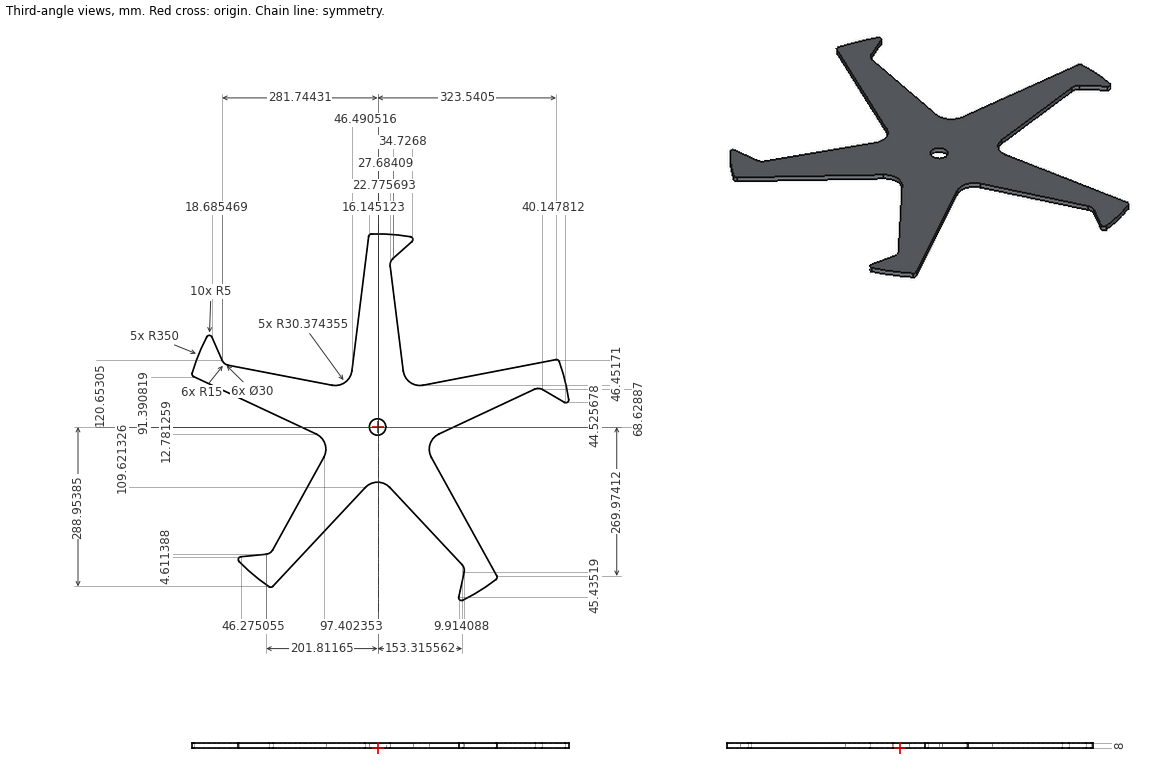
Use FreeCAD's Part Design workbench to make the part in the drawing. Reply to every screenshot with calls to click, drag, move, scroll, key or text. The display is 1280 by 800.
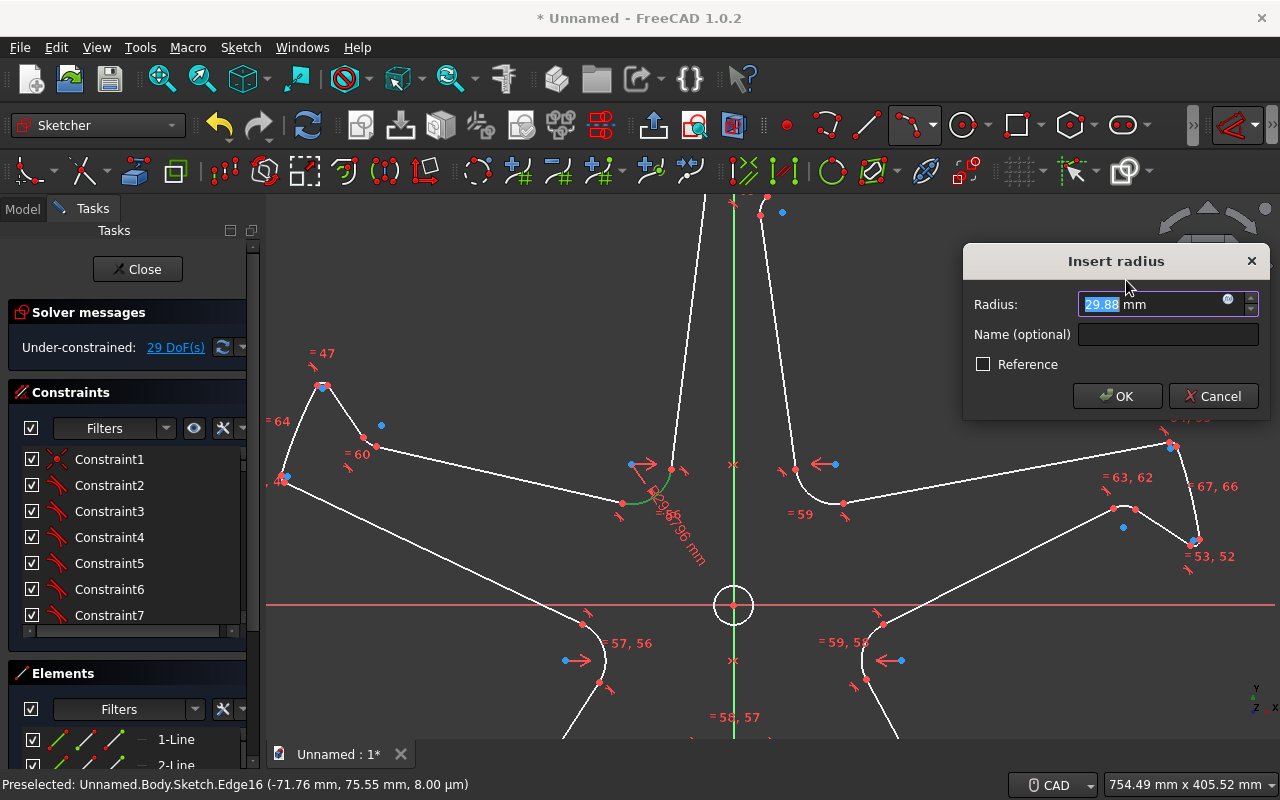
text(30.374355)
key(Return)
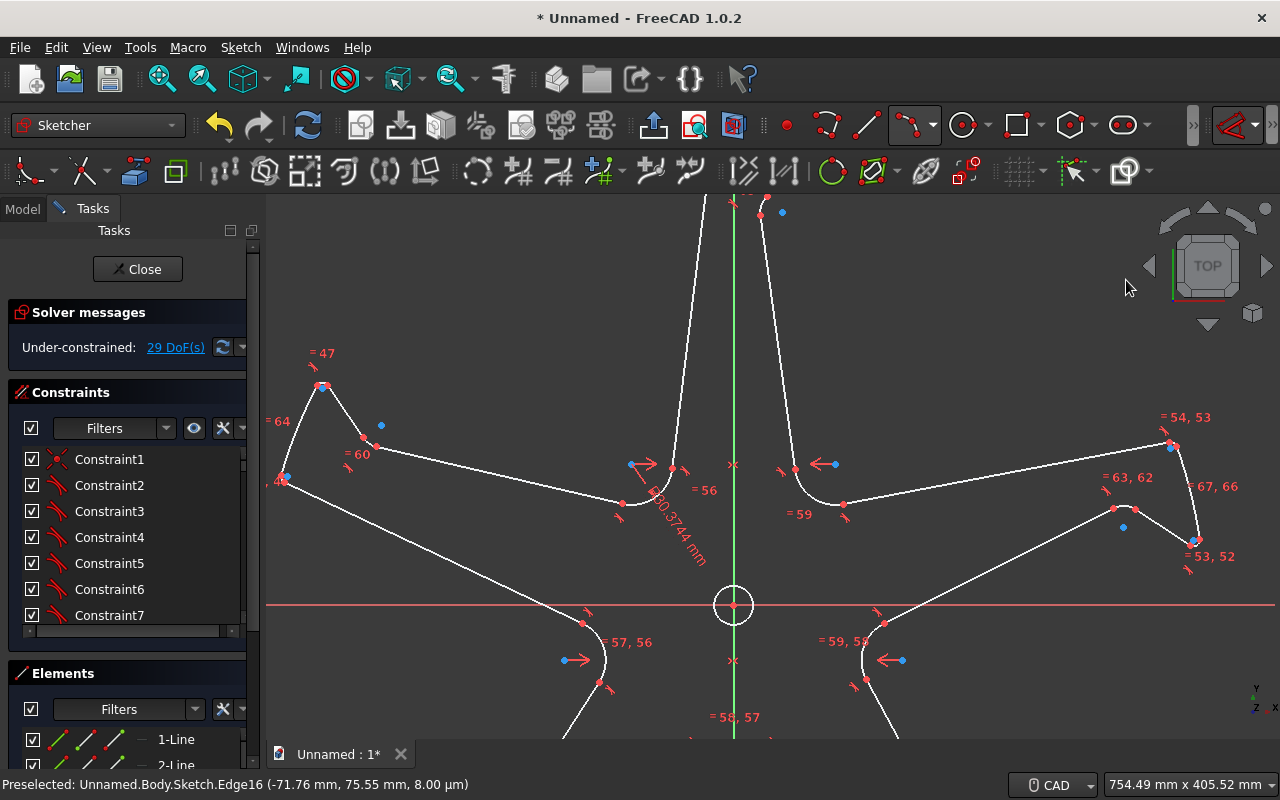
scroll(369, 444, up, 4)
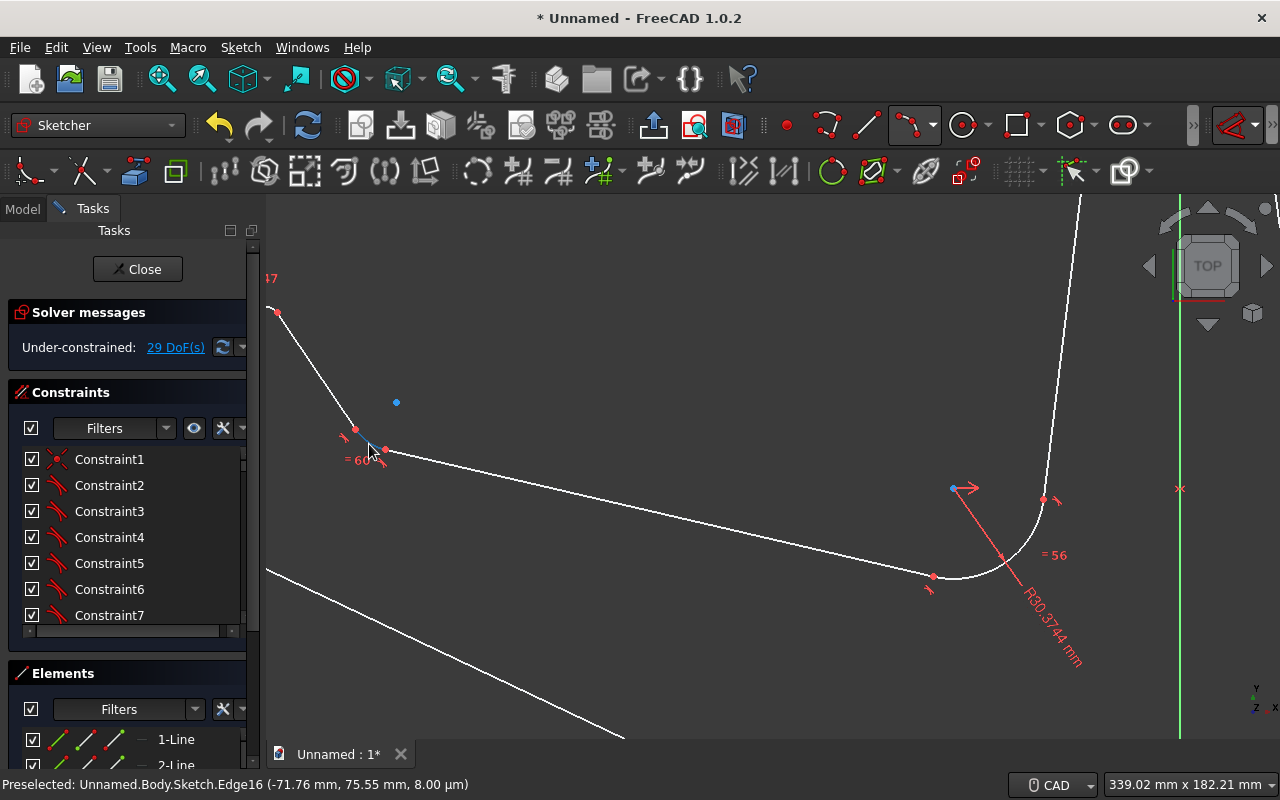
click(369, 442)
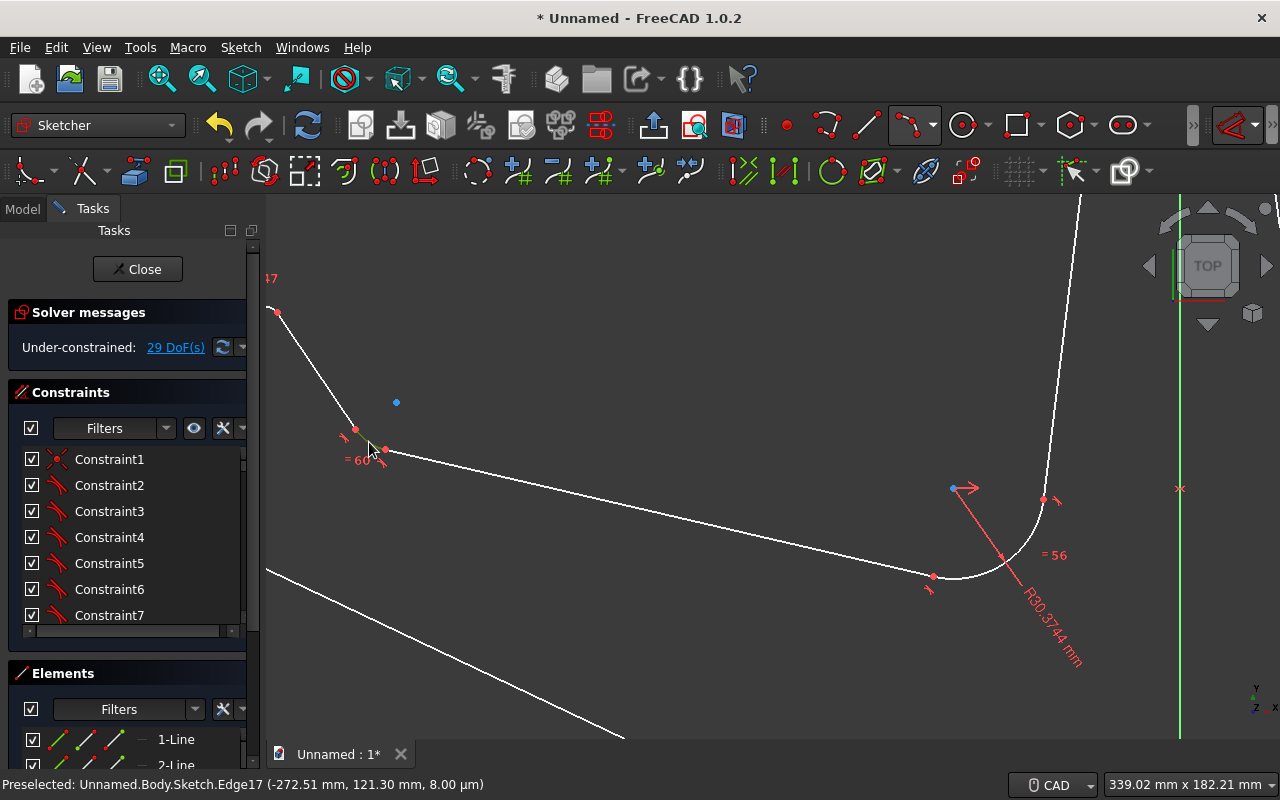
key(k)
key(r)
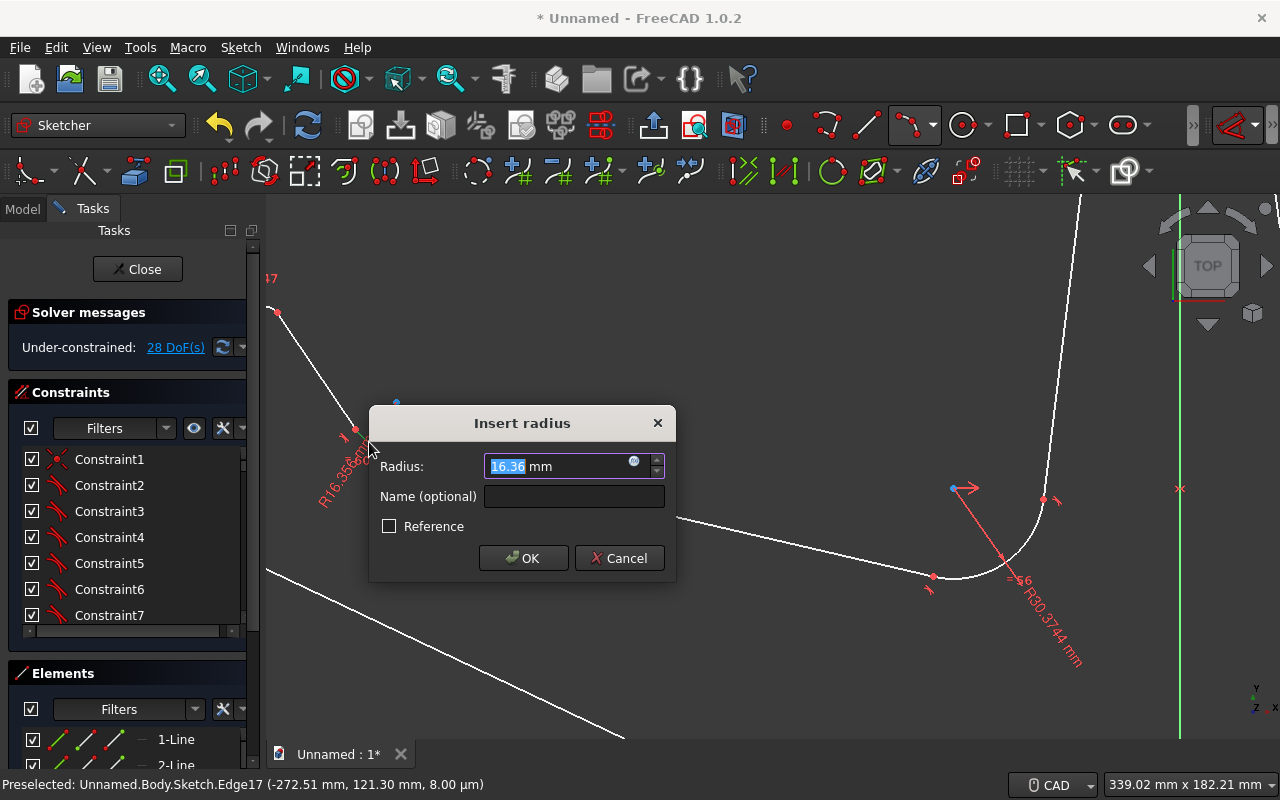
text(15)
key(Return)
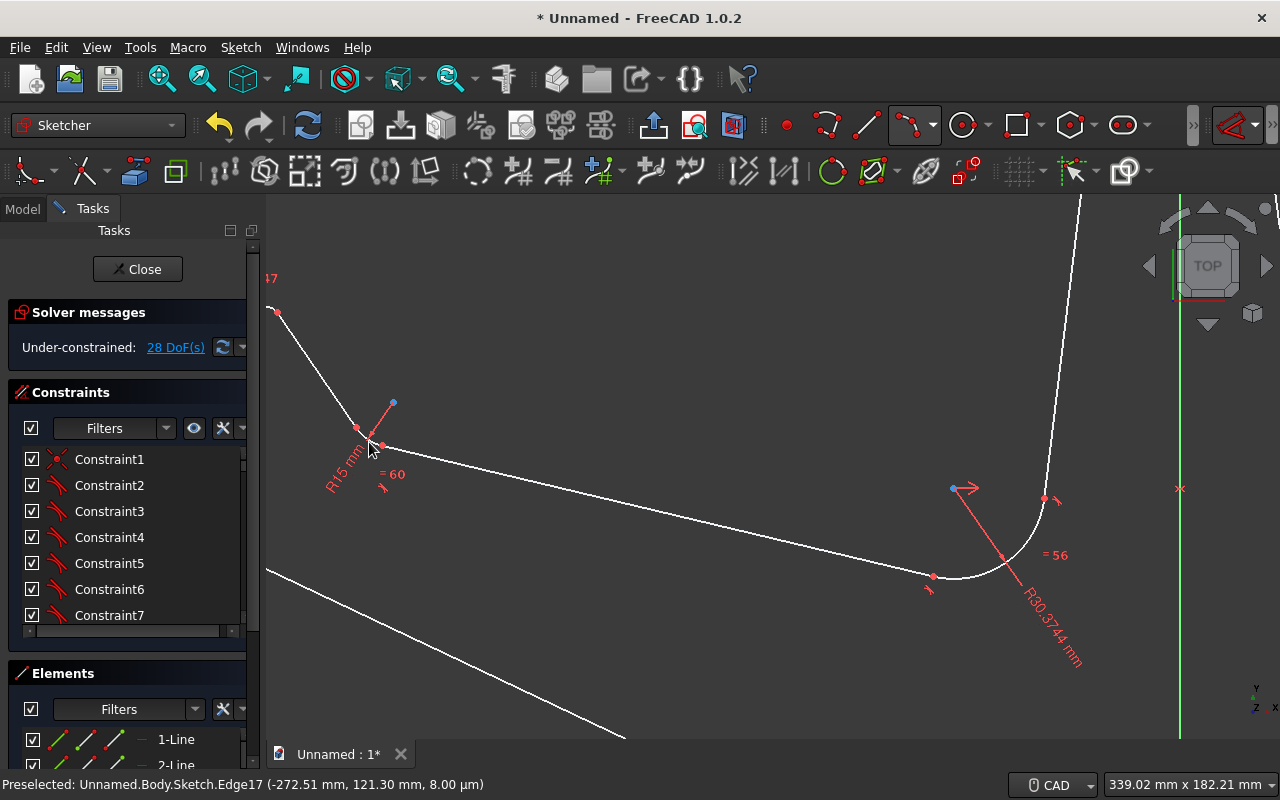
scroll(607, 410, down, 9)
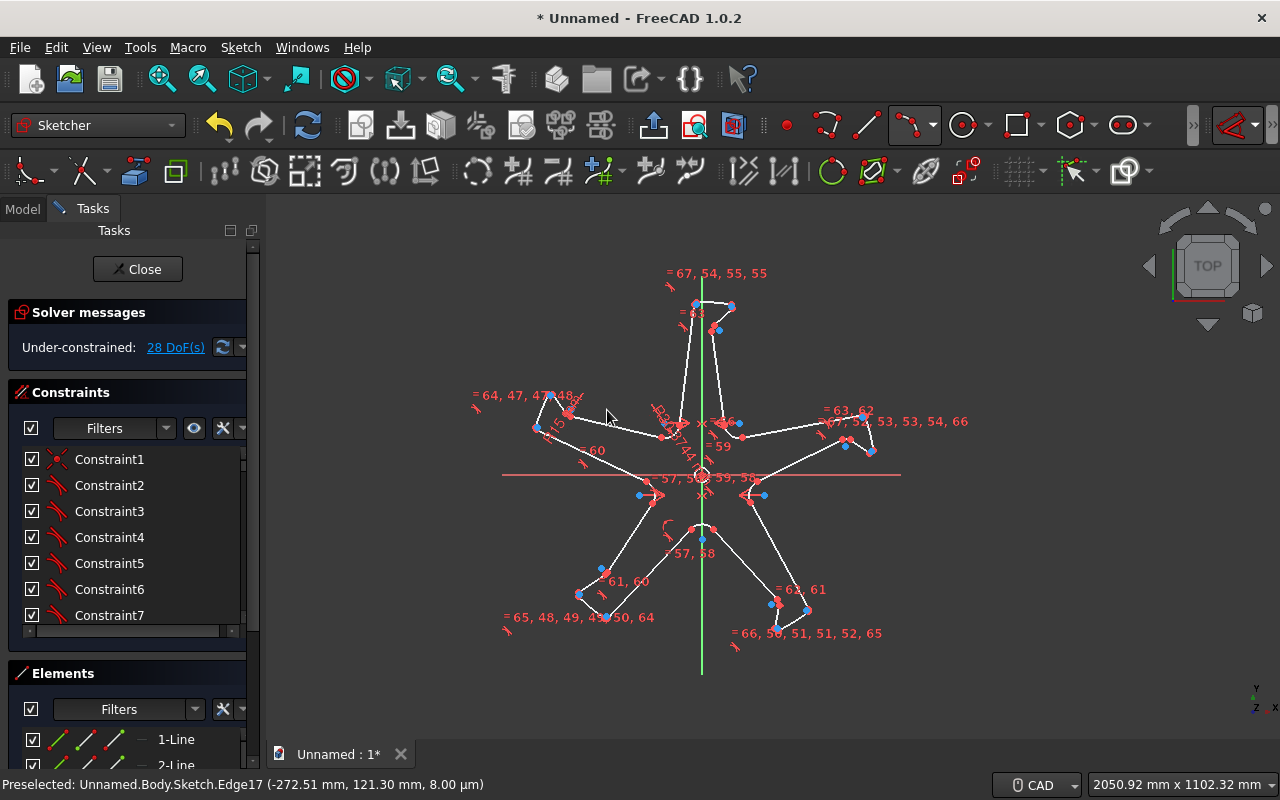
scroll(551, 393, up, 14)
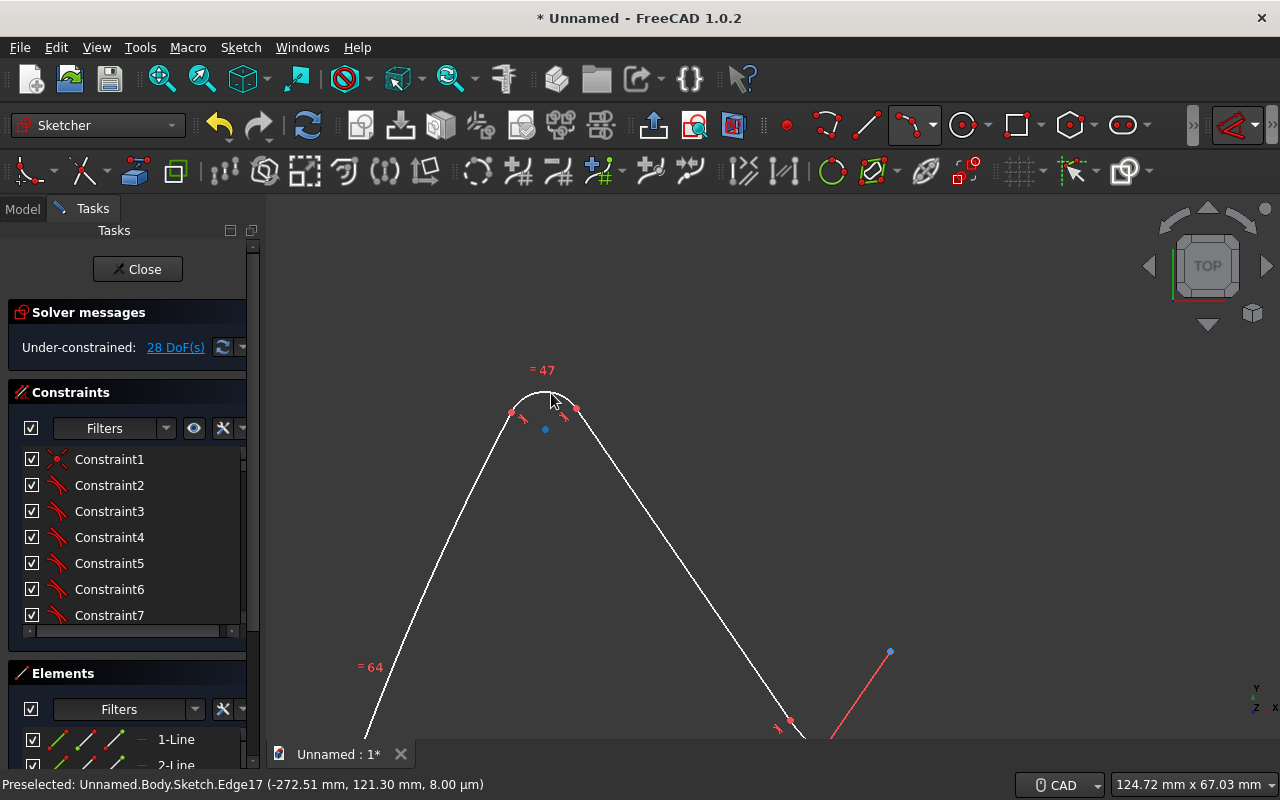
click(543, 392)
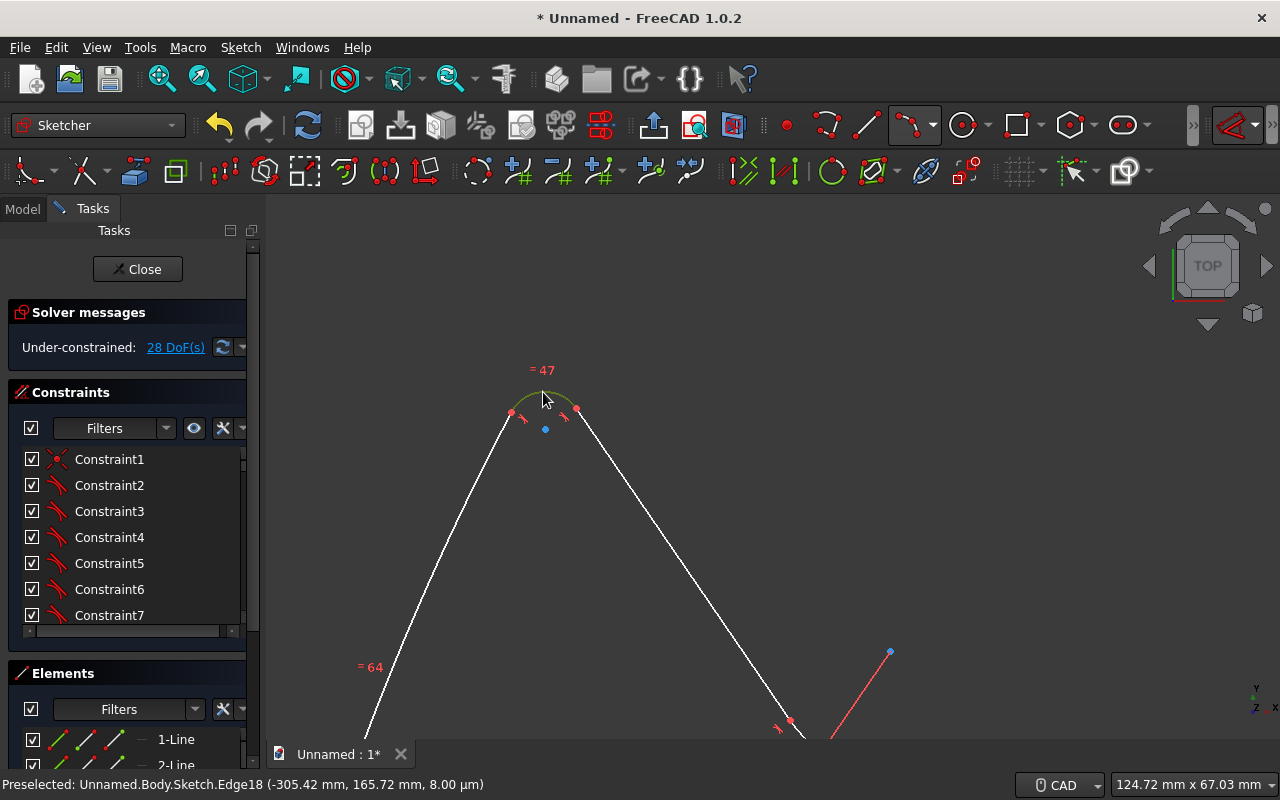
click(1258, 126)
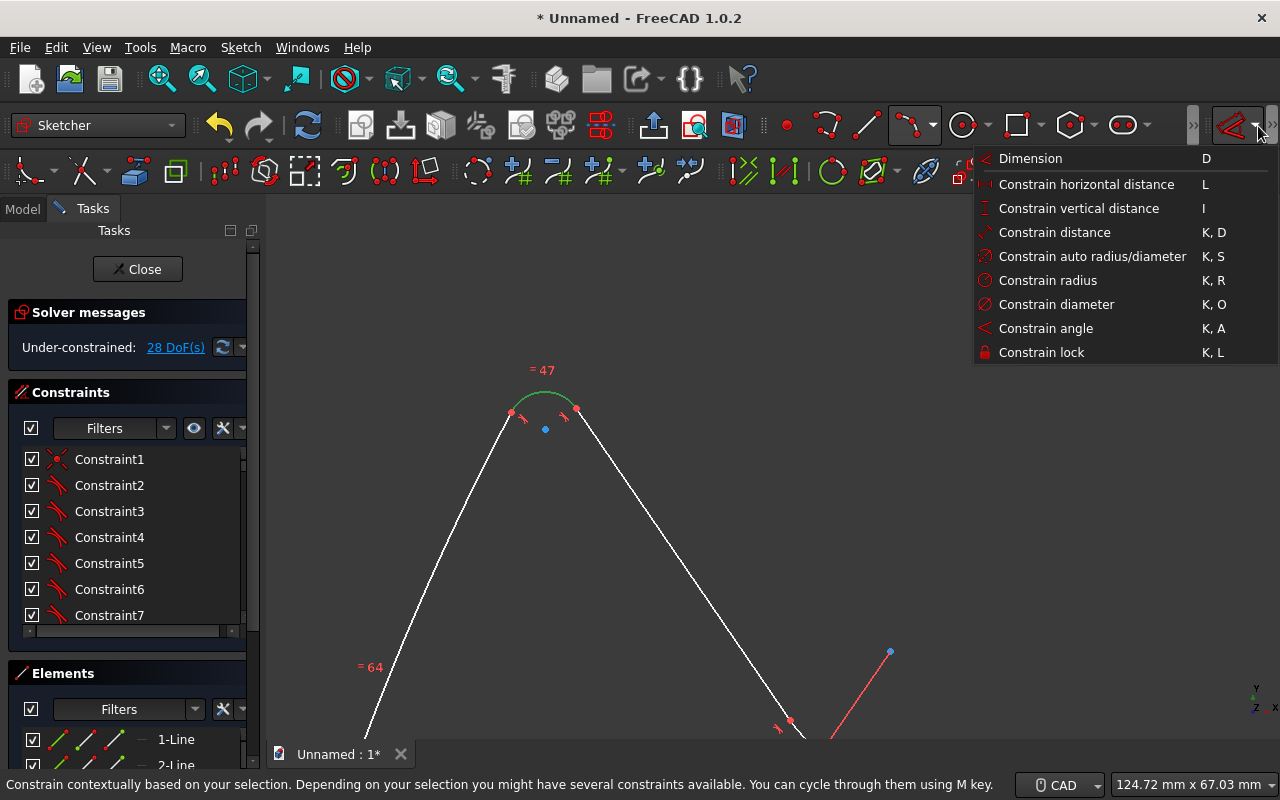
click(1126, 280)